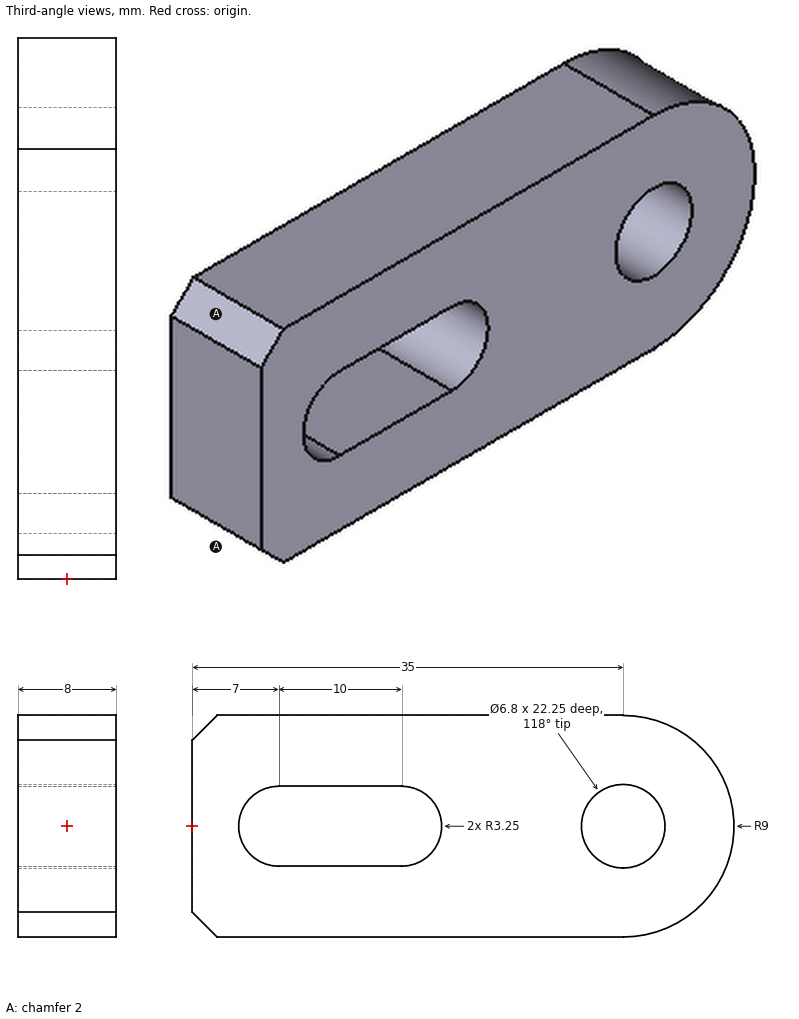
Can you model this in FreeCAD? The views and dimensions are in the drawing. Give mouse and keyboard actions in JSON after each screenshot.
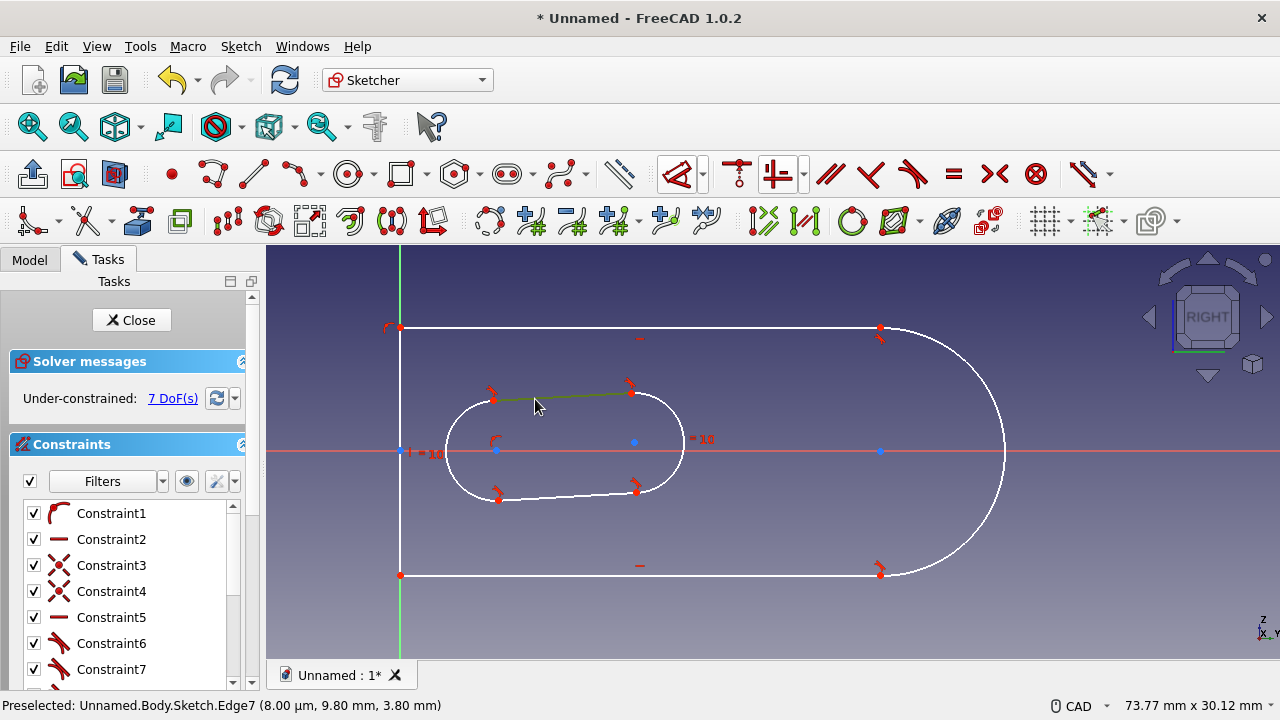
{"action": "key", "text": "h"}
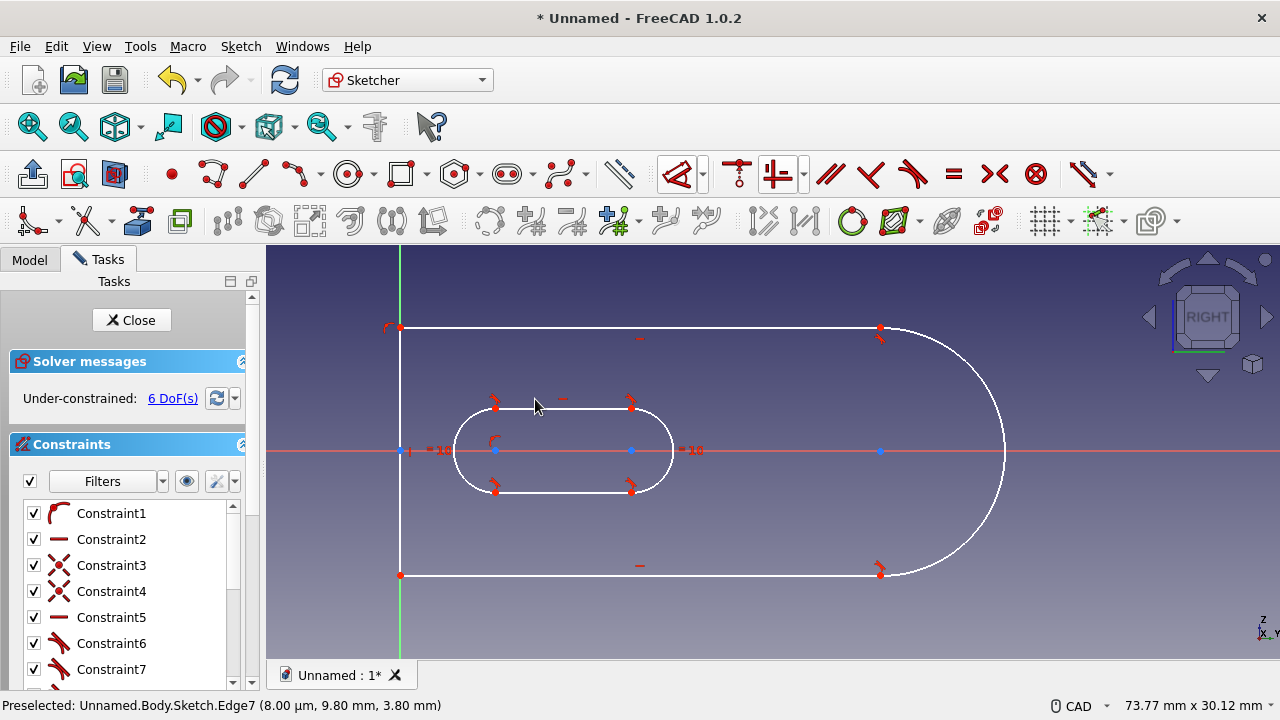
{"action": "left_click", "coordinate": [881, 452]}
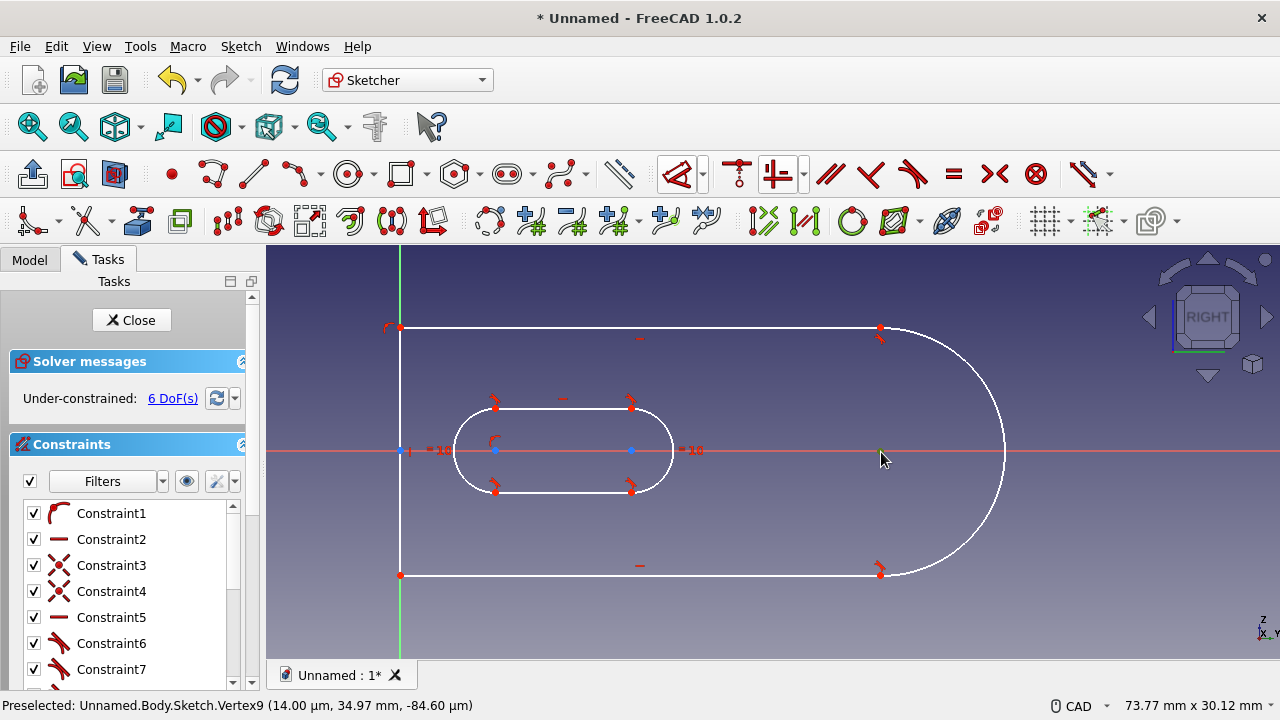
{"action": "left_click", "coordinate": [353, 451]}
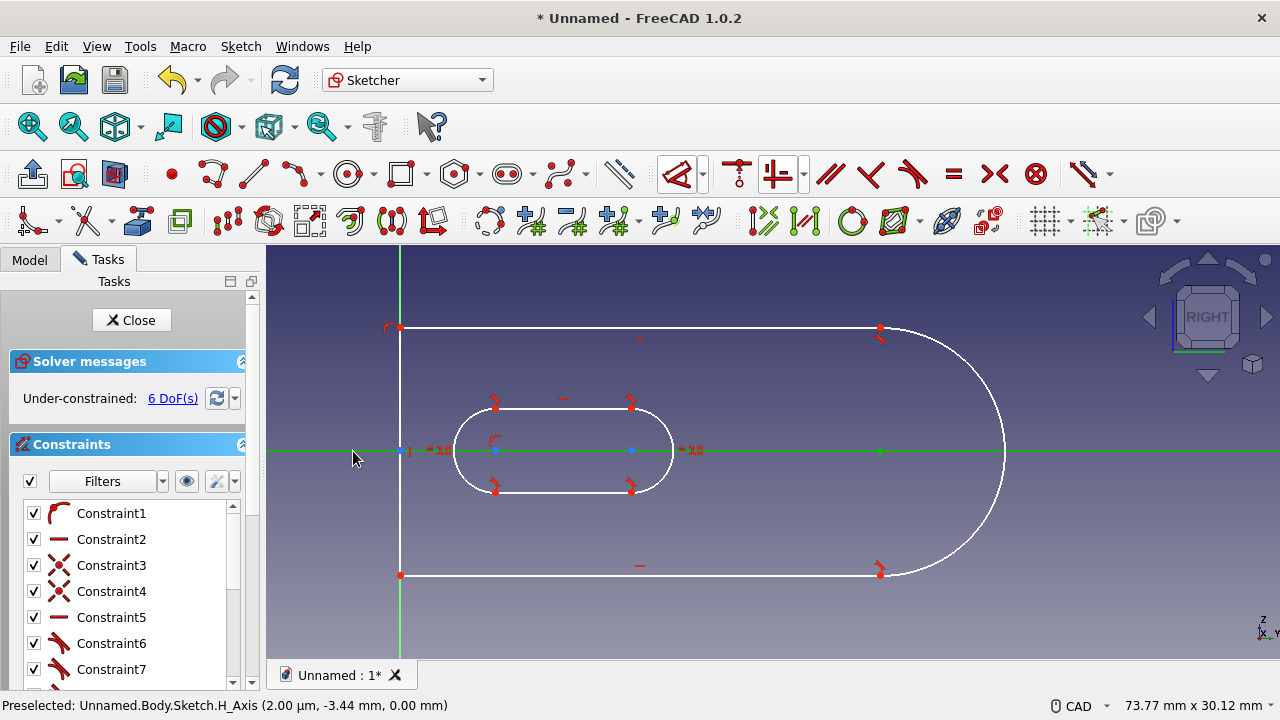
{"action": "left_click", "coordinate": [737, 174]}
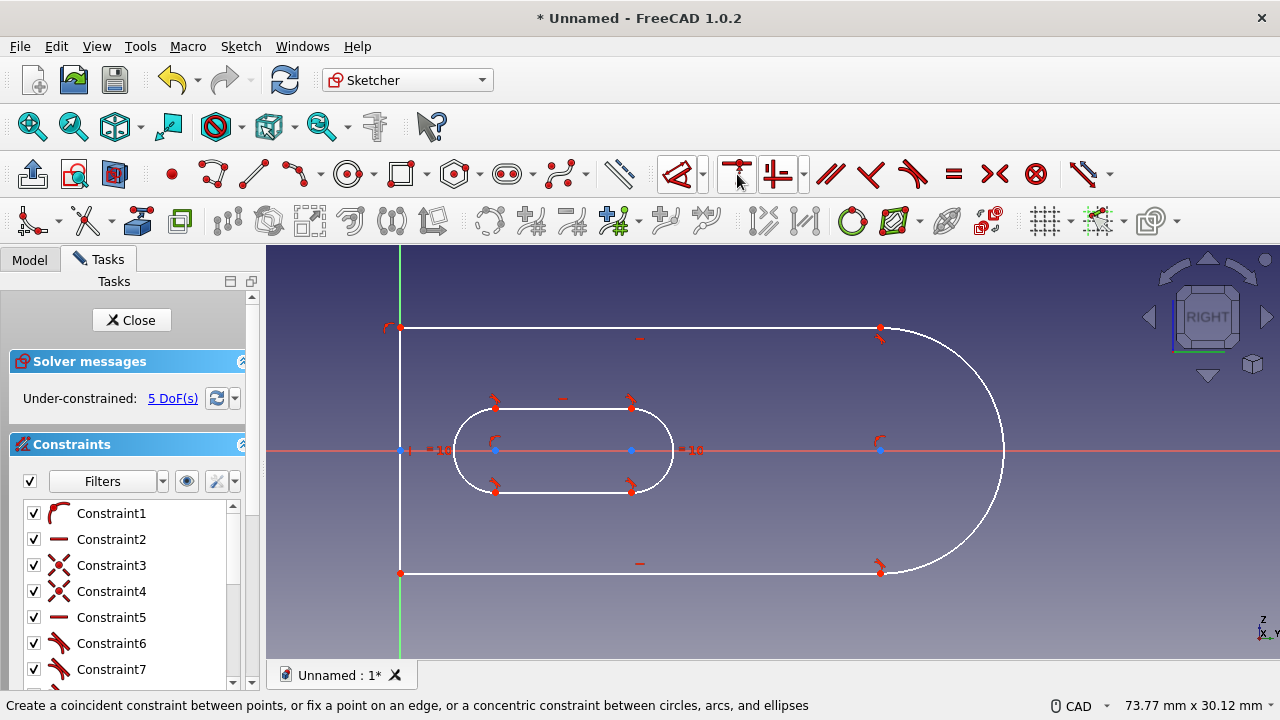
{"action": "left_click", "coordinate": [676, 174]}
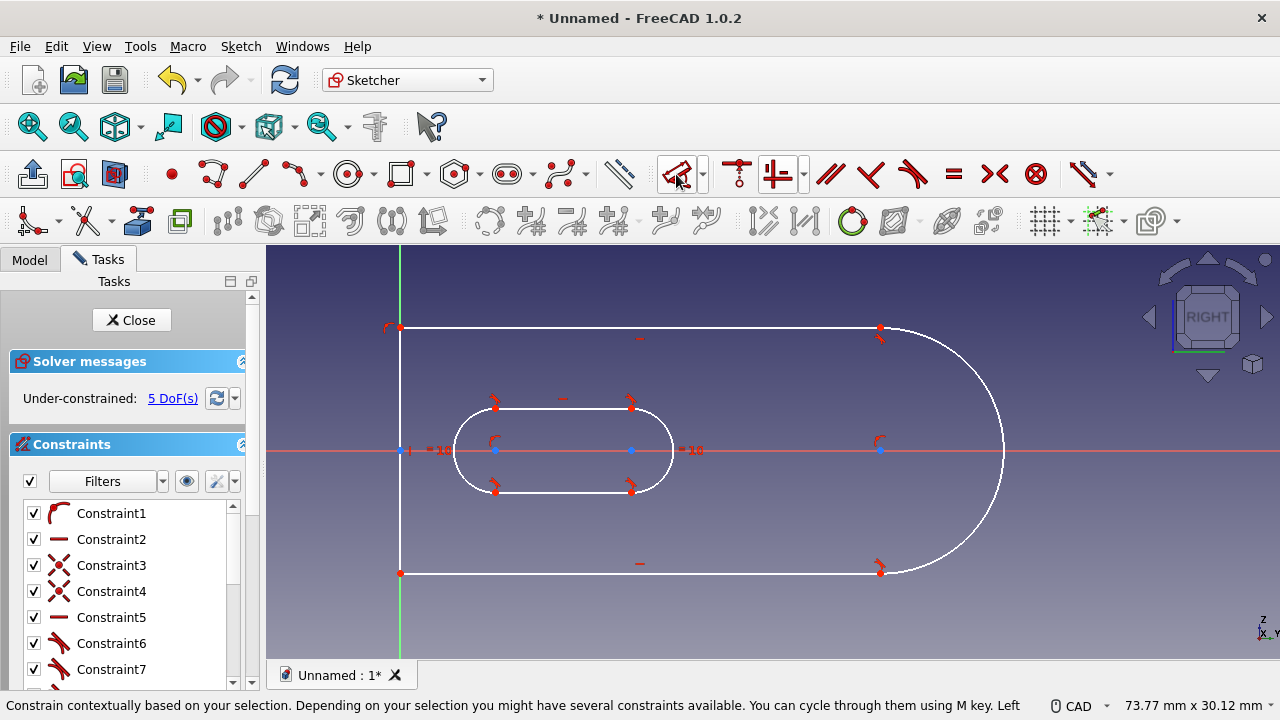
{"action": "left_click", "coordinate": [980, 523]}
{"action": "left_click", "coordinate": [1006, 542]}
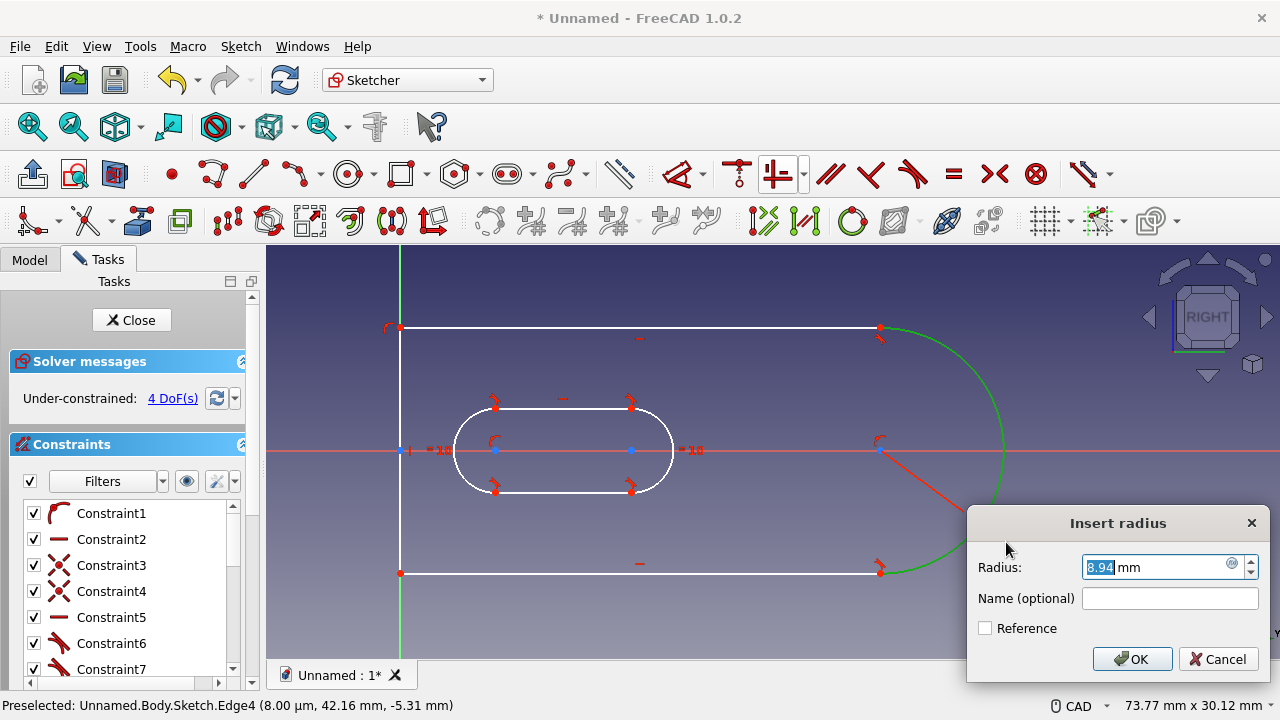
{"action": "type", "text": "9"}
{"action": "key", "text": "Return"}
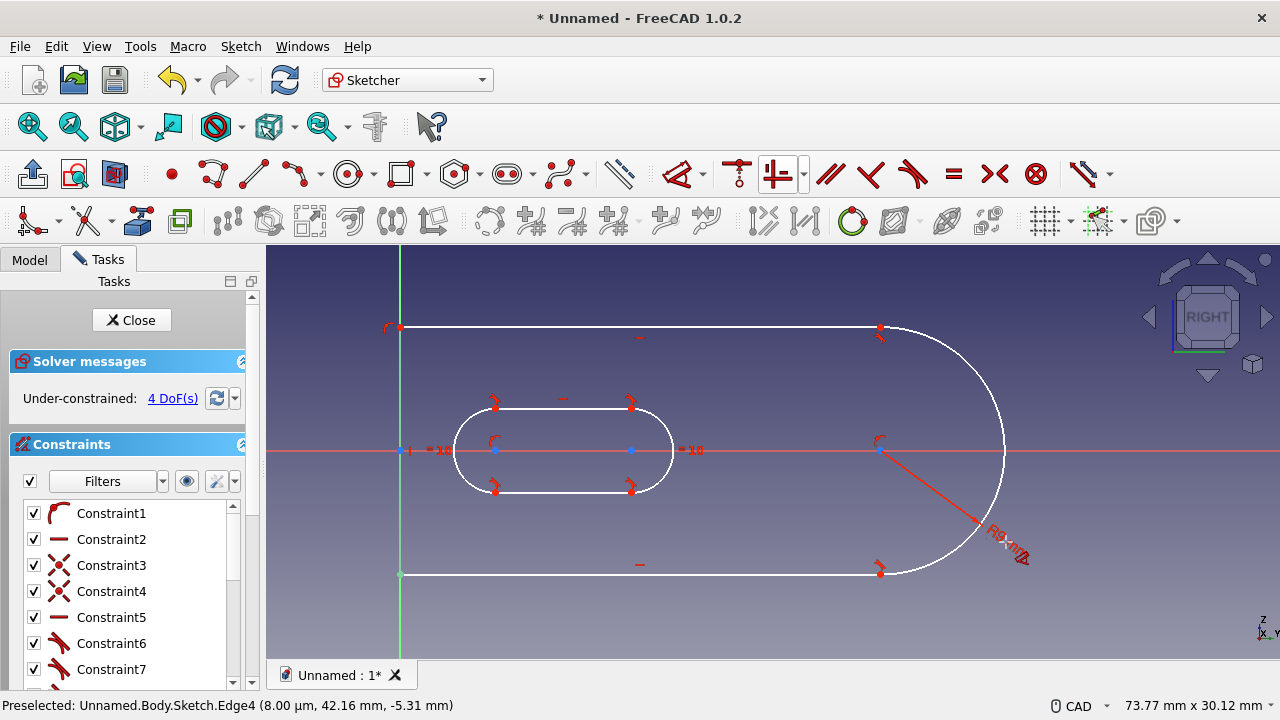
{"action": "left_click", "coordinate": [462, 426]}
{"action": "left_click", "coordinate": [436, 407]}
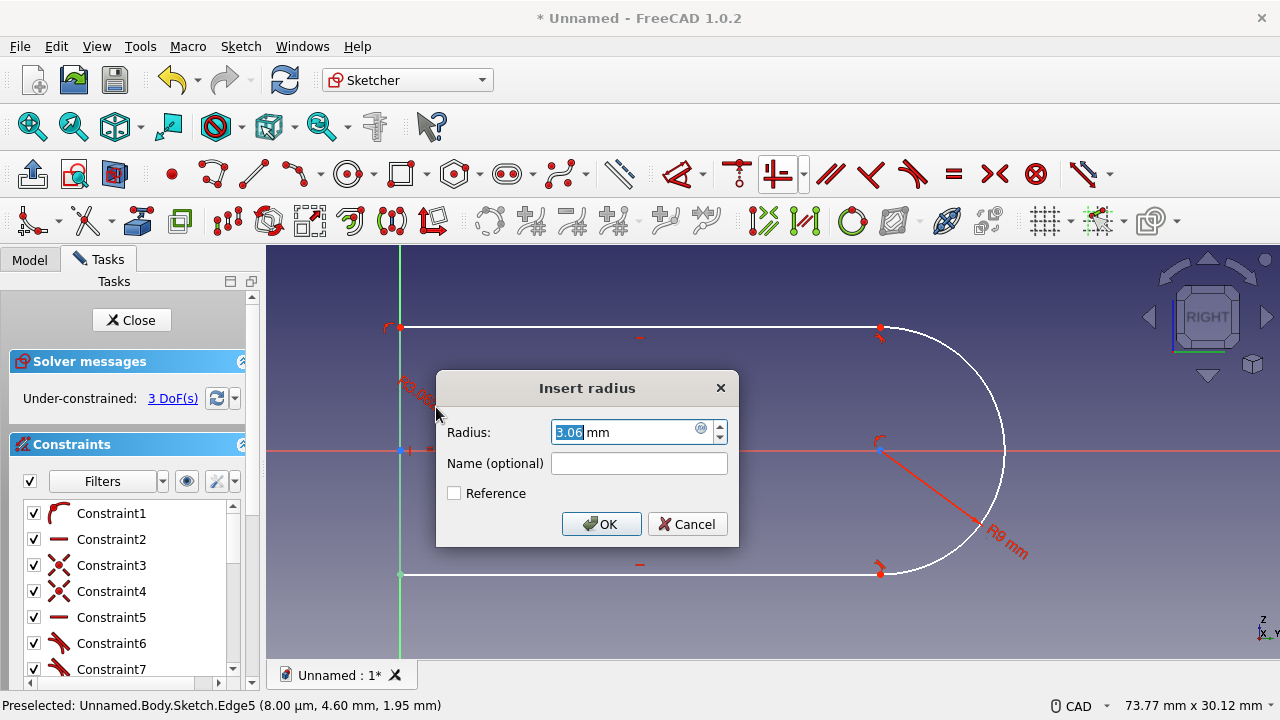
{"action": "type", "text": "3.25"}
{"action": "key", "text": "Return"}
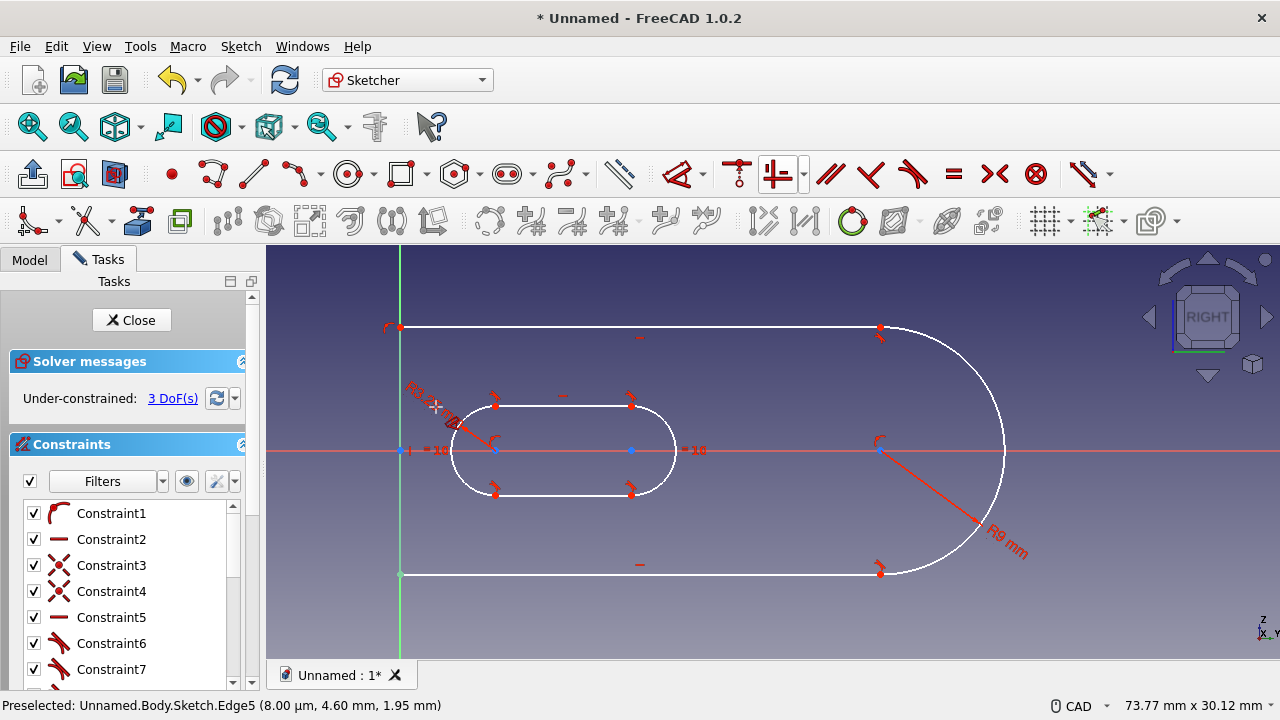
{"action": "left_click", "coordinate": [737, 327]}
{"action": "left_click", "coordinate": [641, 293]}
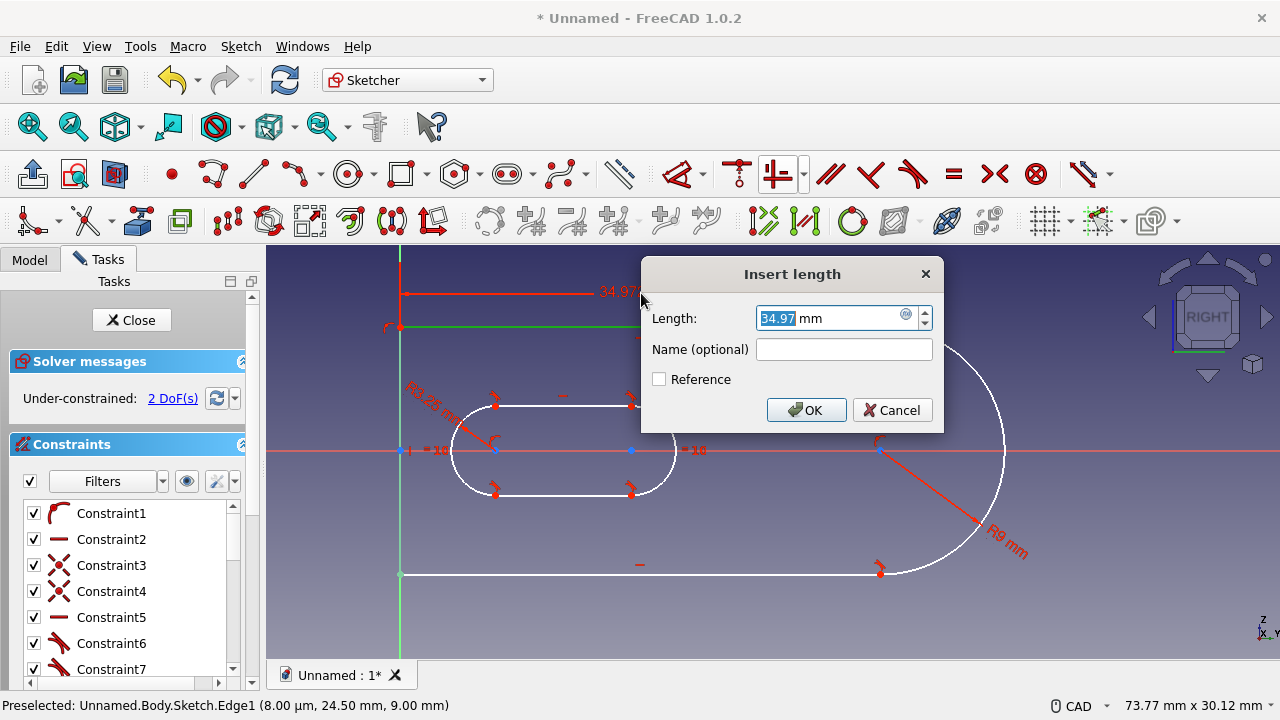
{"action": "type", "text": "35"}
{"action": "key", "text": "Return"}